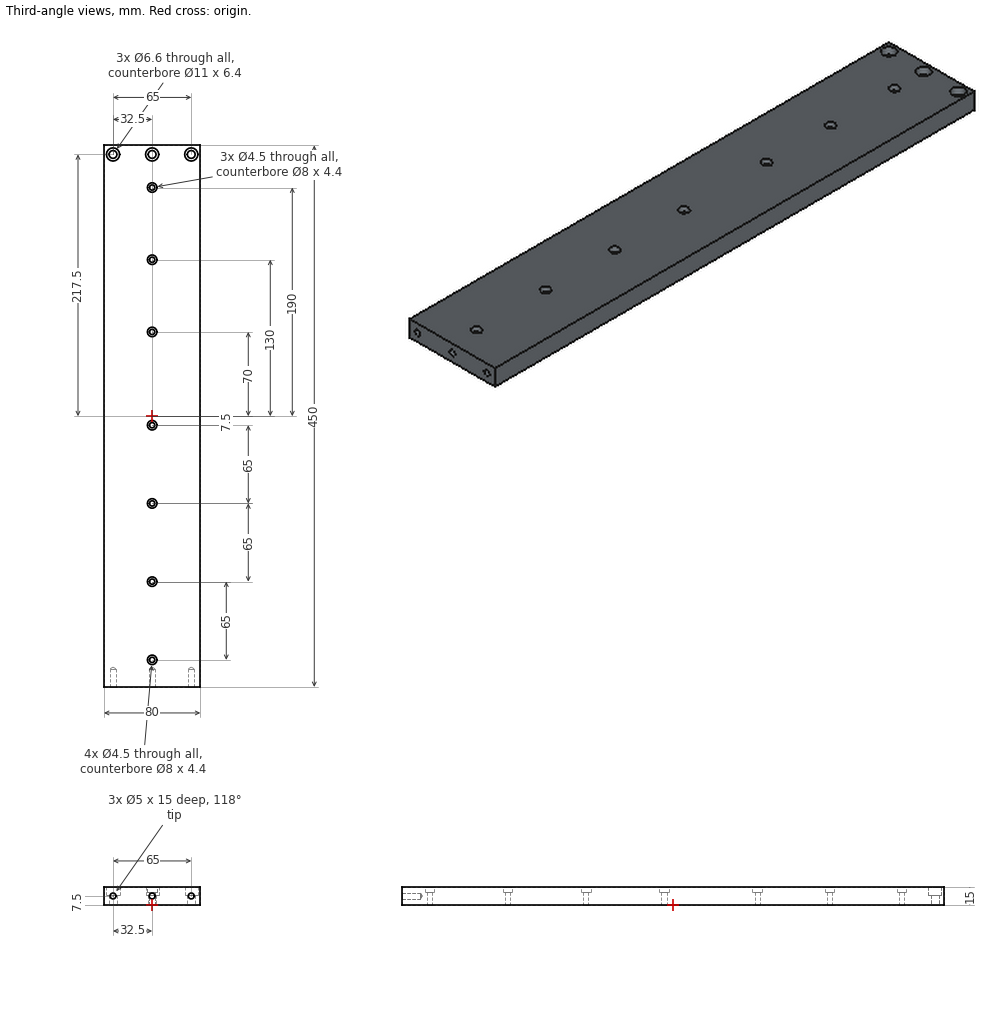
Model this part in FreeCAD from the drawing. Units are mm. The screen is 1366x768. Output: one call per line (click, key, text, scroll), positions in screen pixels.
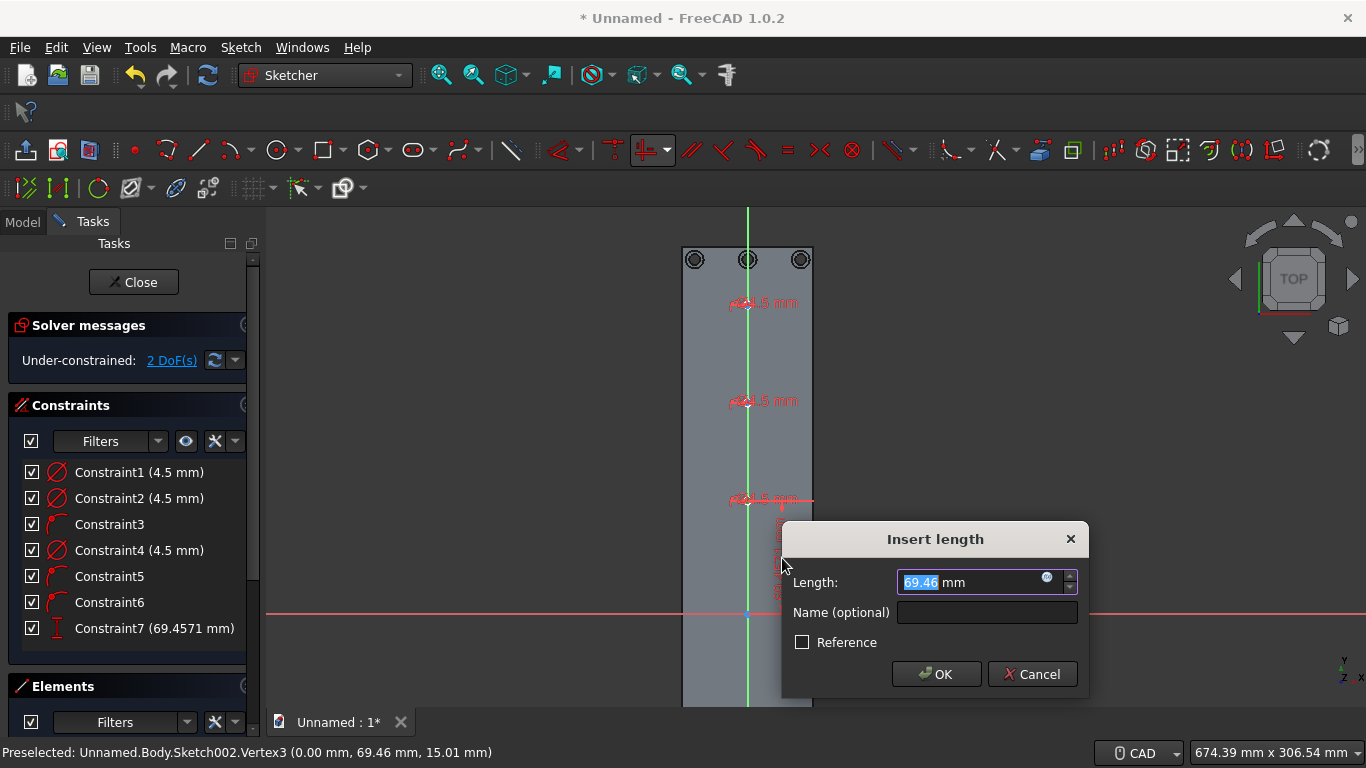
text(70)
key(Return)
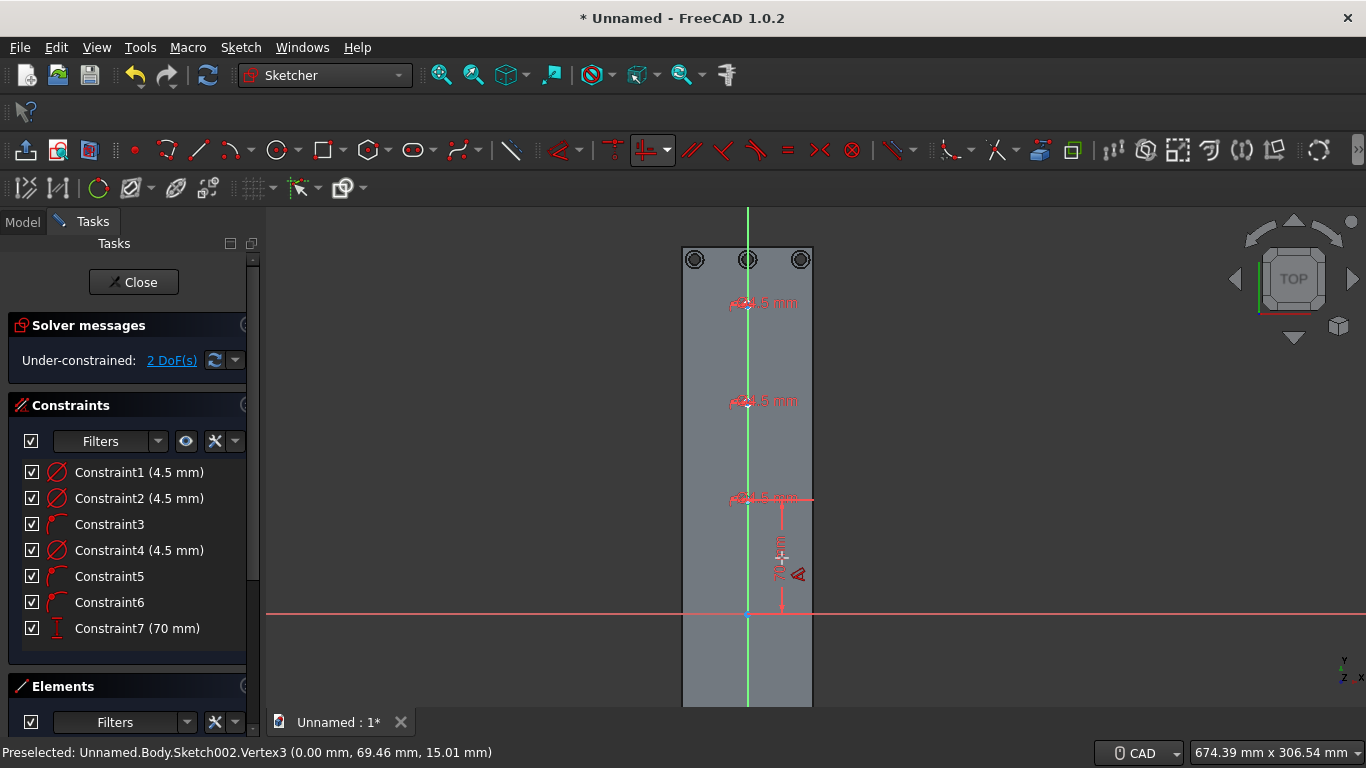
click(748, 305)
click(782, 460)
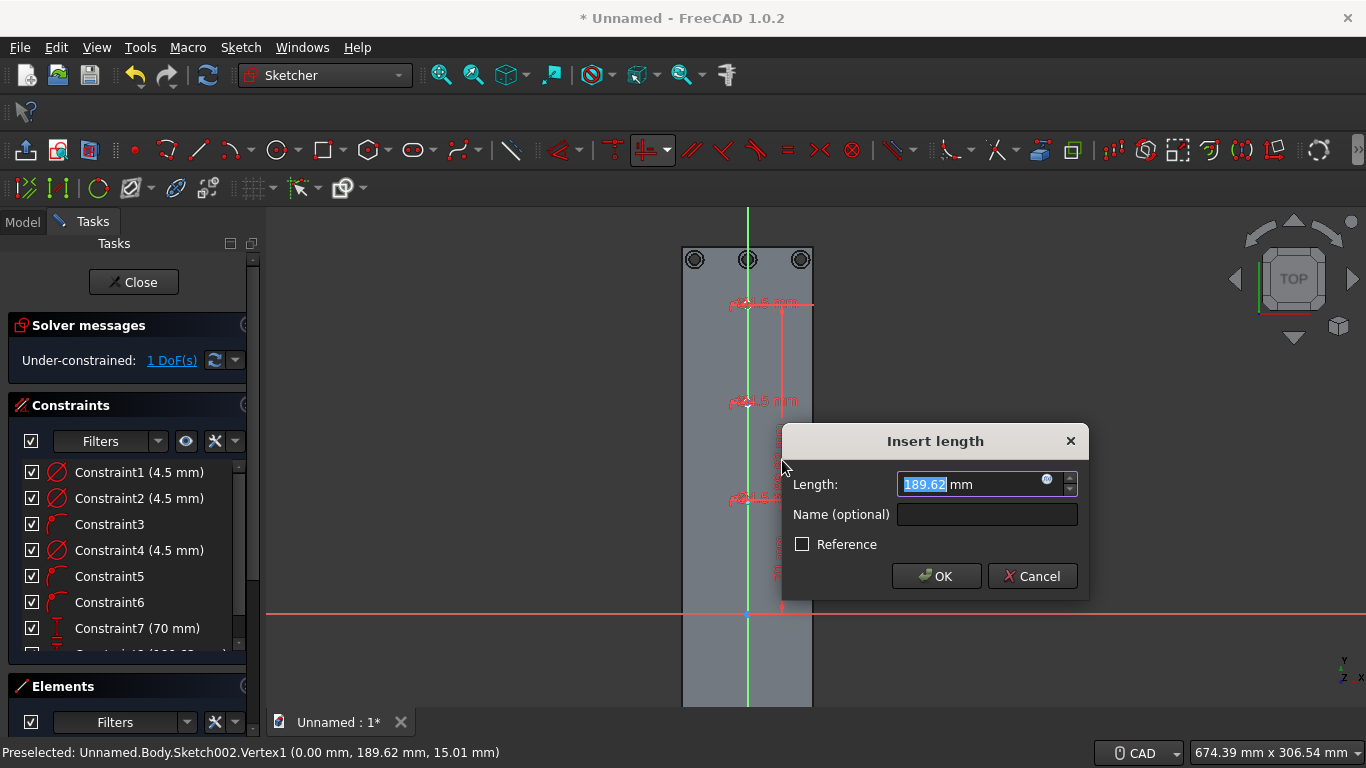
text(190)
key(Return)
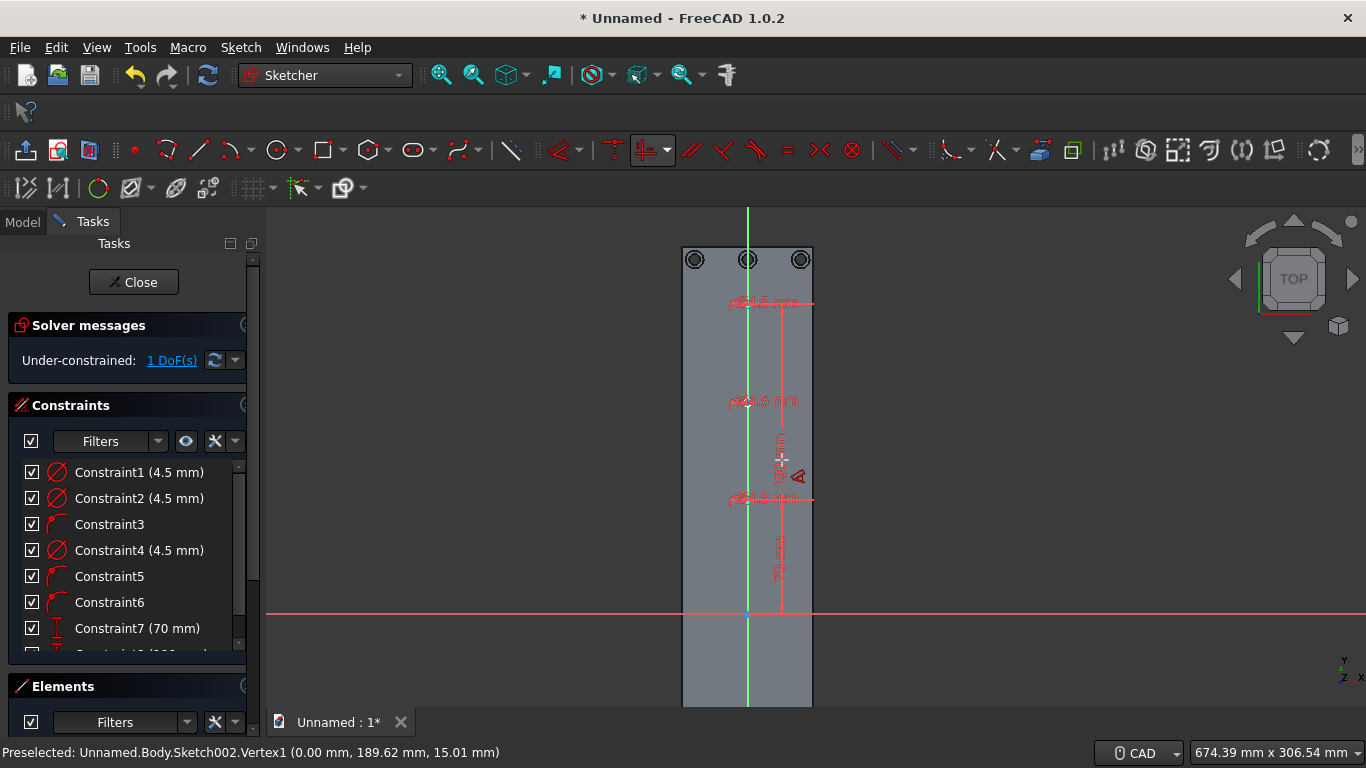
click(748, 403)
click(782, 509)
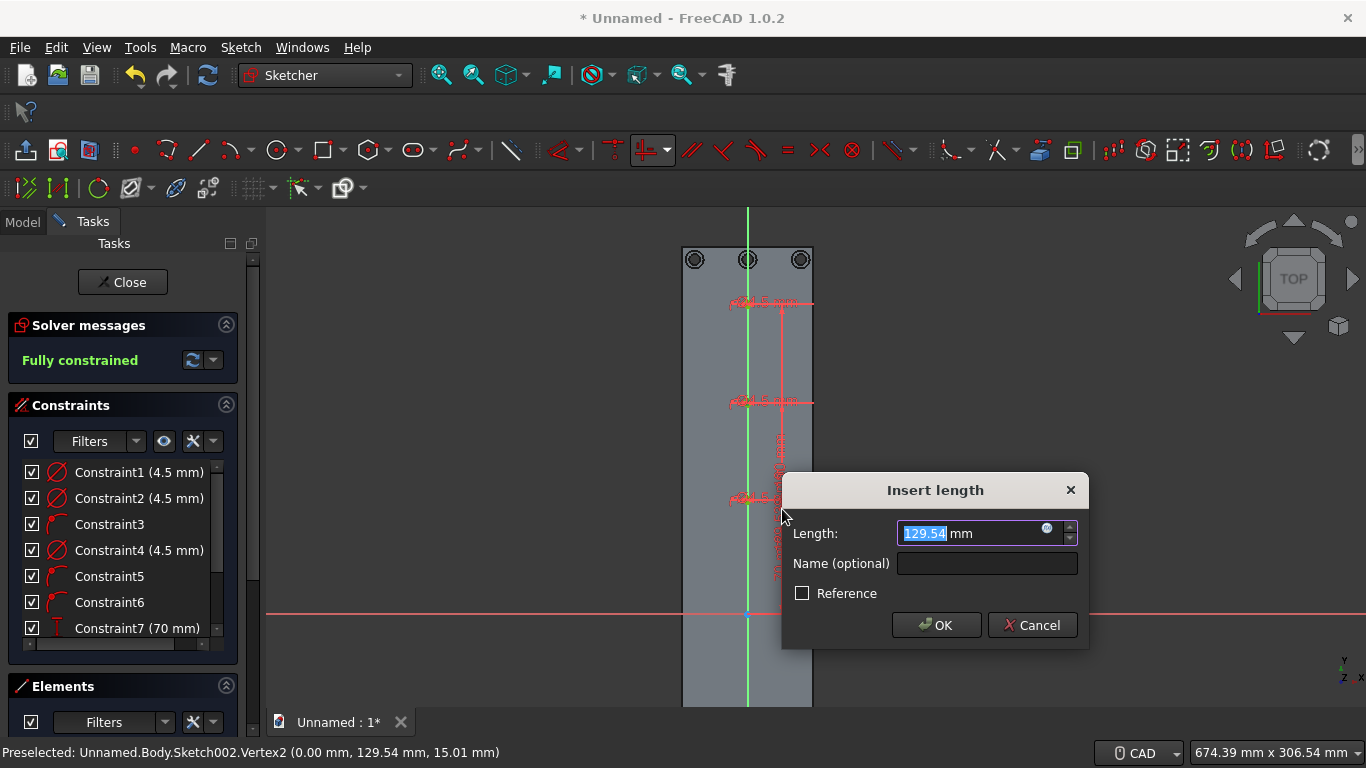
text(130)
key(Return)
key(Escape)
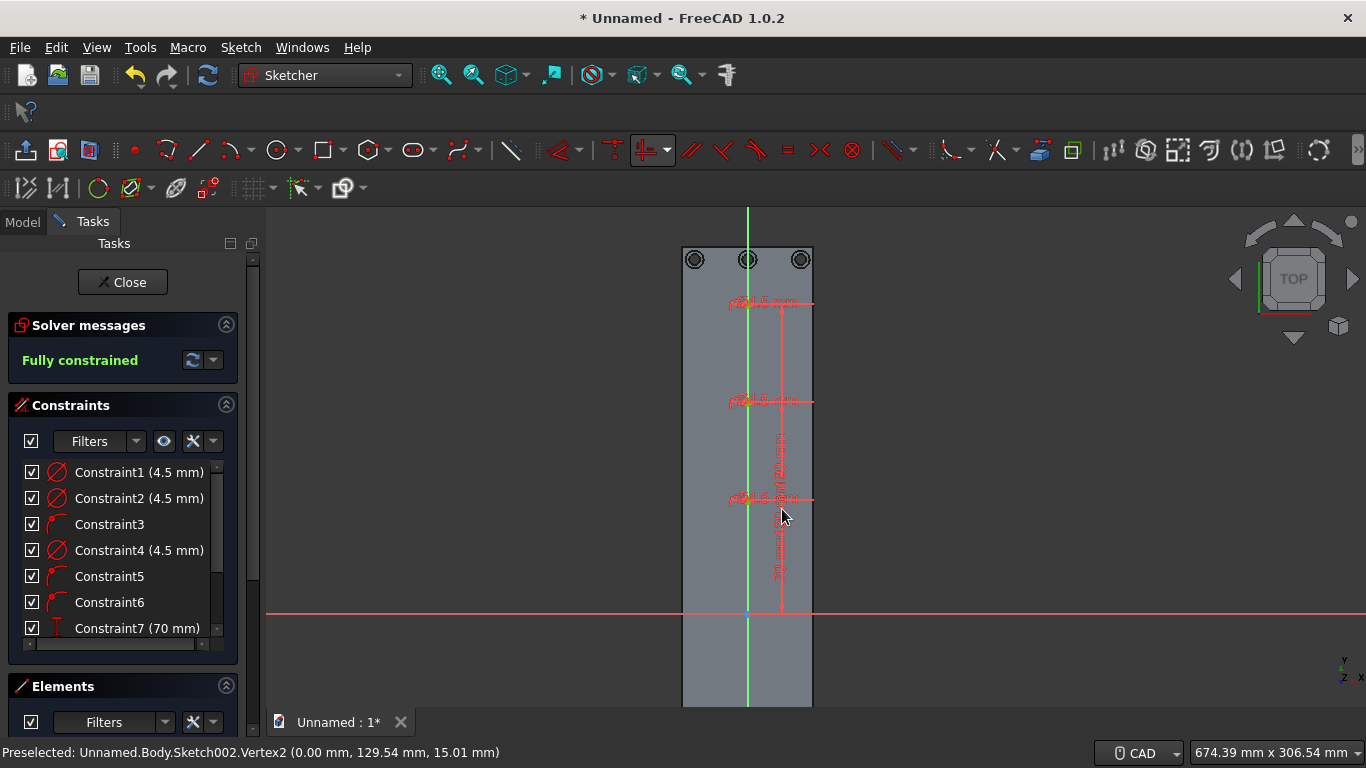
click(123, 282)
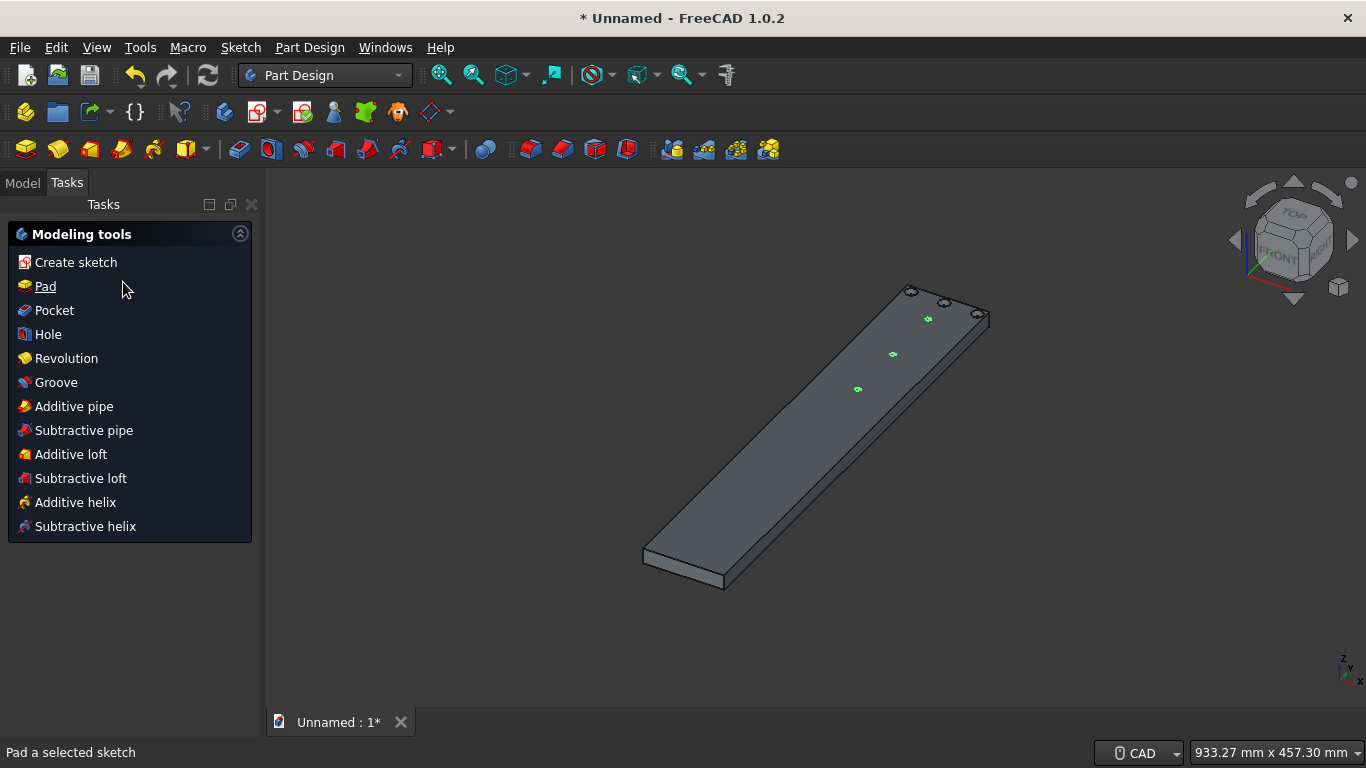
click(272, 150)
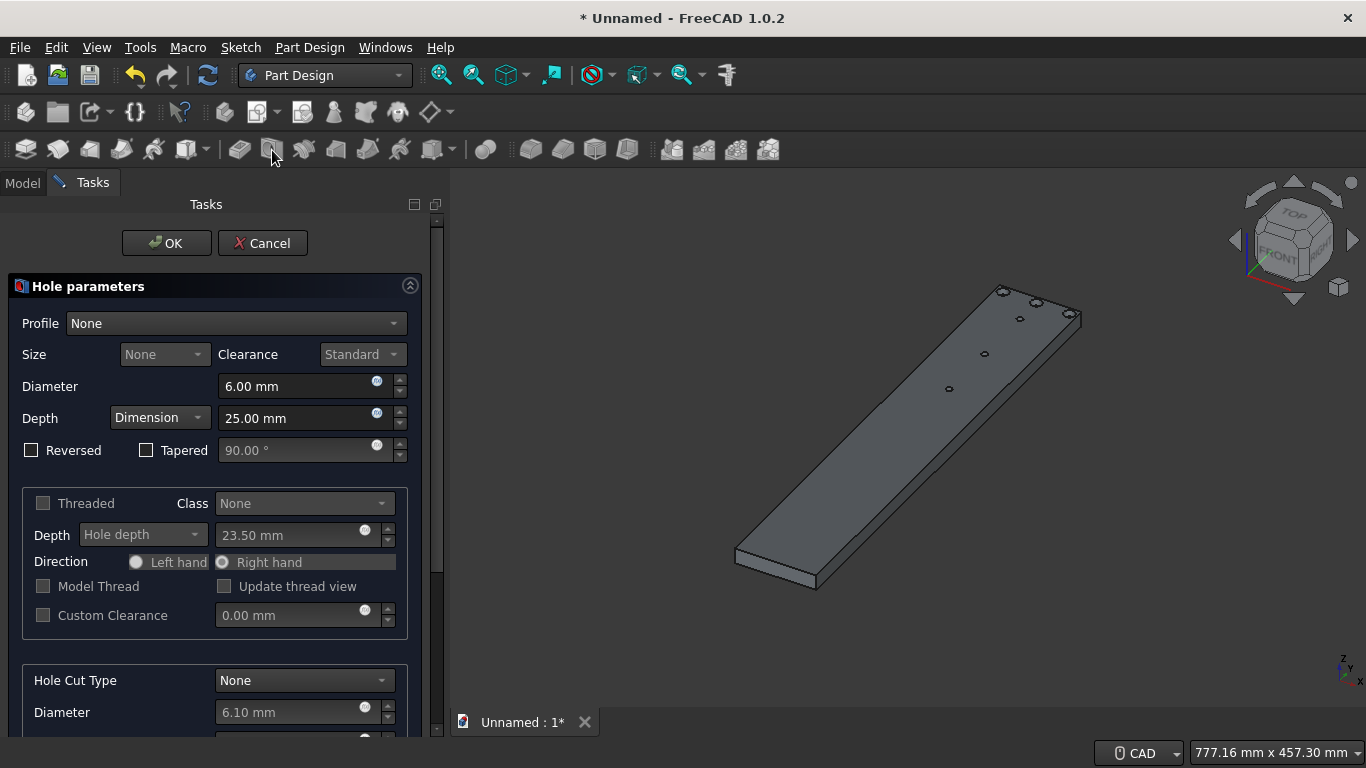
triple_click(305, 386)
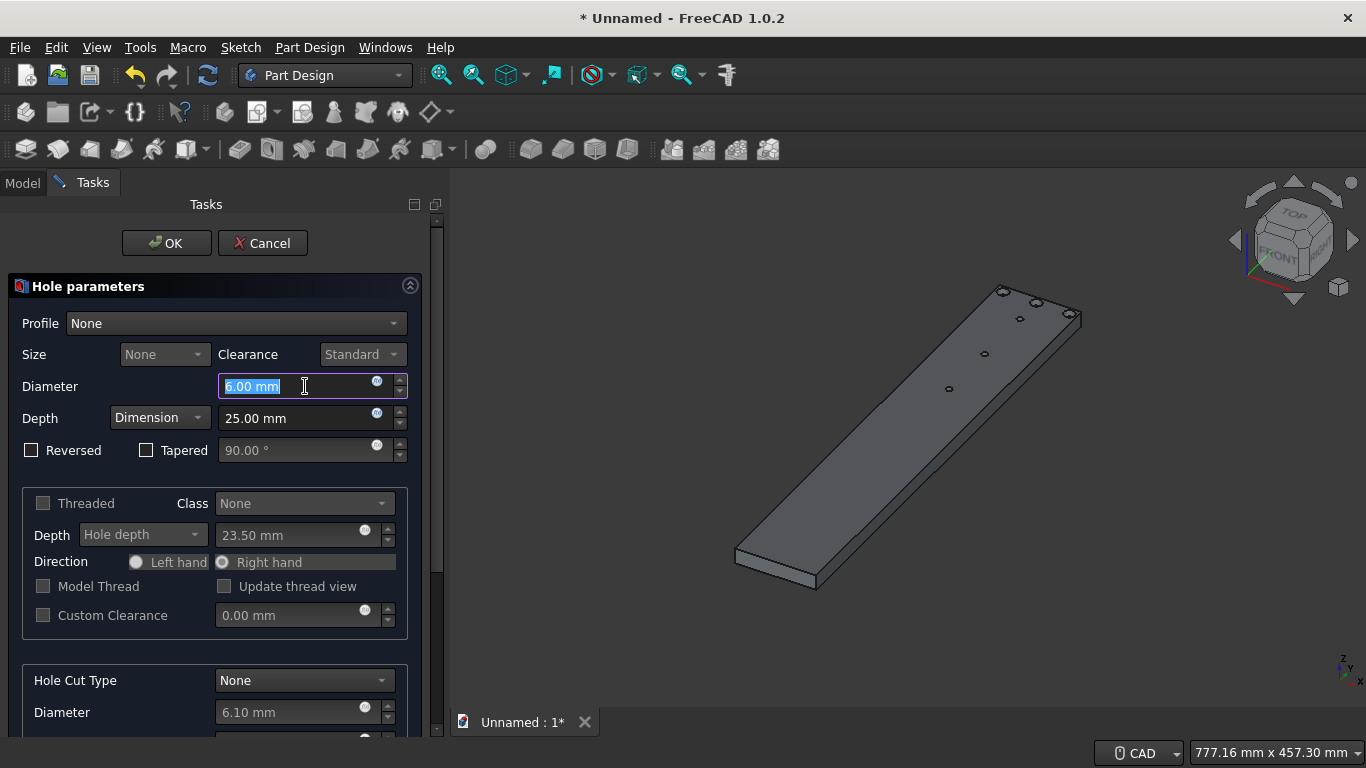
text(4.5)
key(Tab)